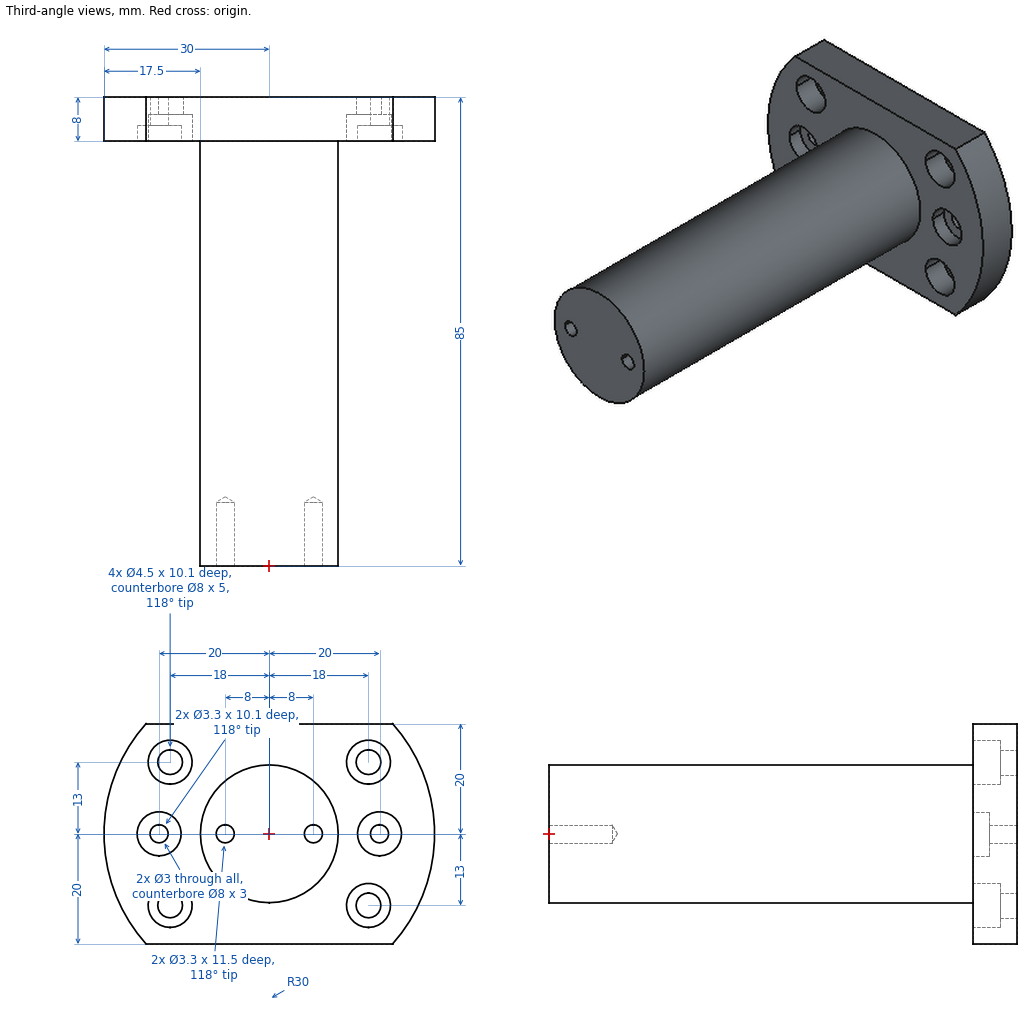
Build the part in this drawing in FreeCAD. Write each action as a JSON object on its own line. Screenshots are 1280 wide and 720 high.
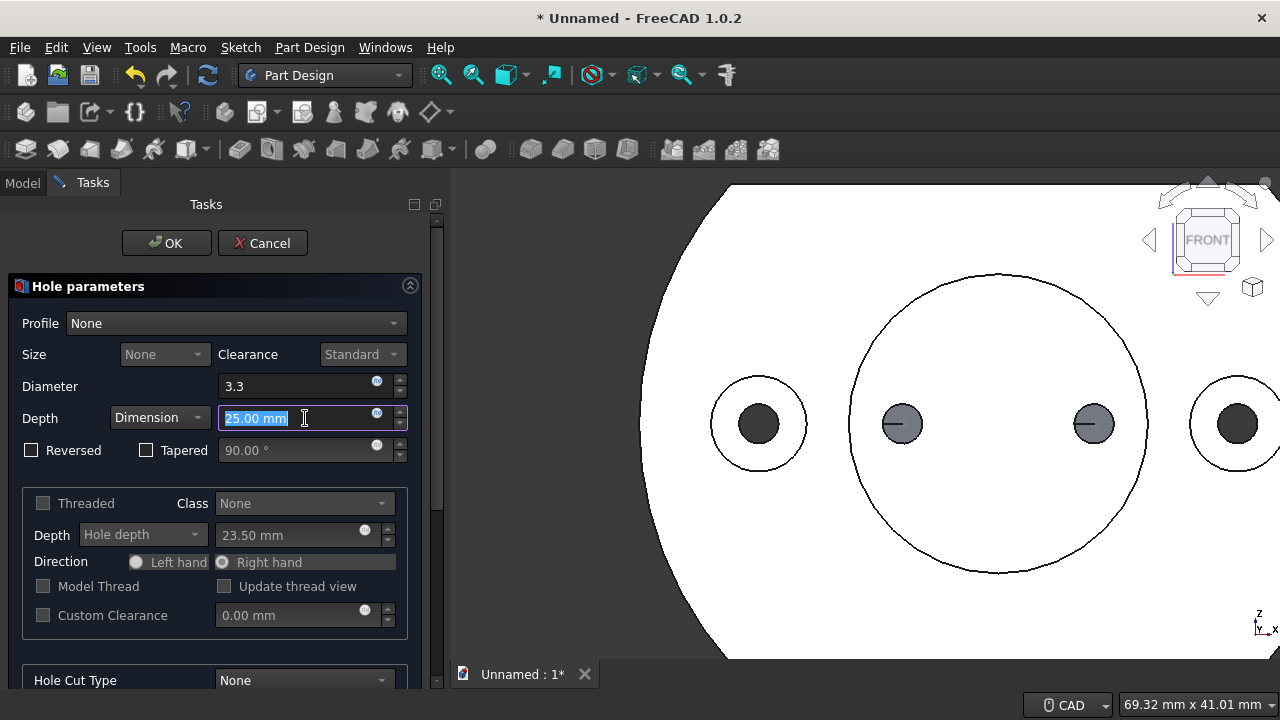
{"action": "type", "text": "10.1"}
{"action": "key", "text": "Tab"}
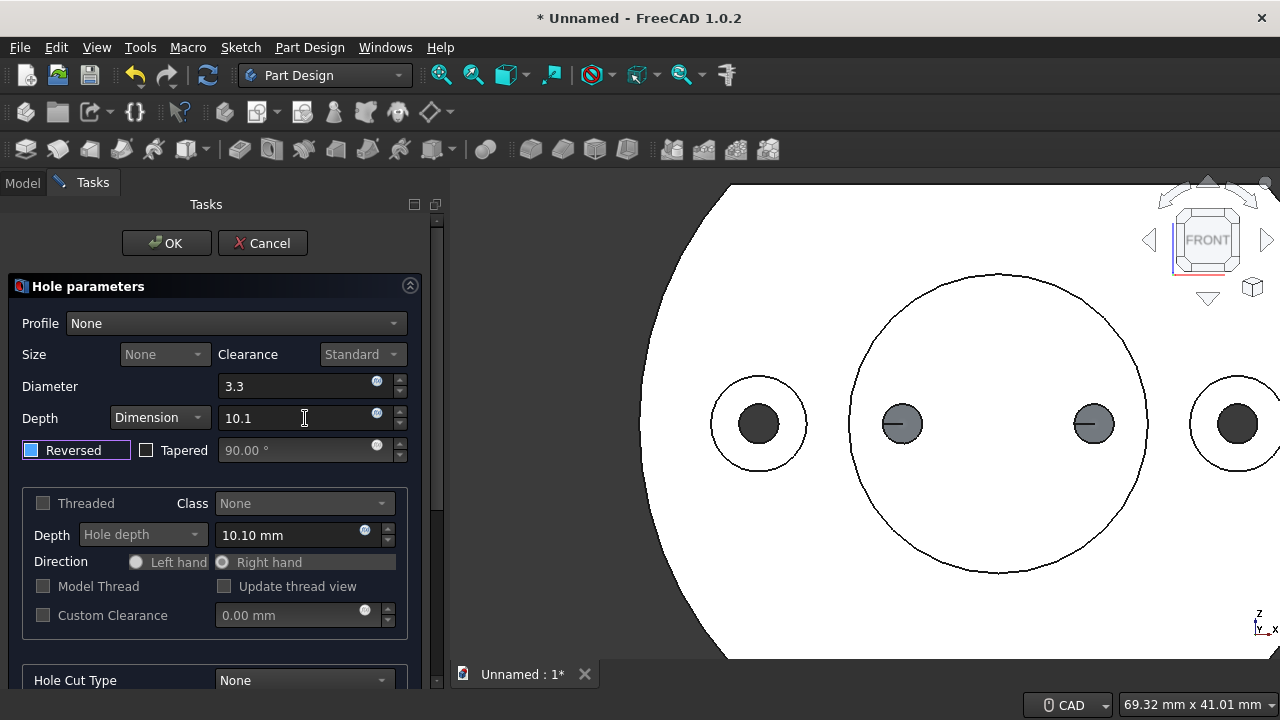
{"action": "left_click", "coordinate": [167, 243]}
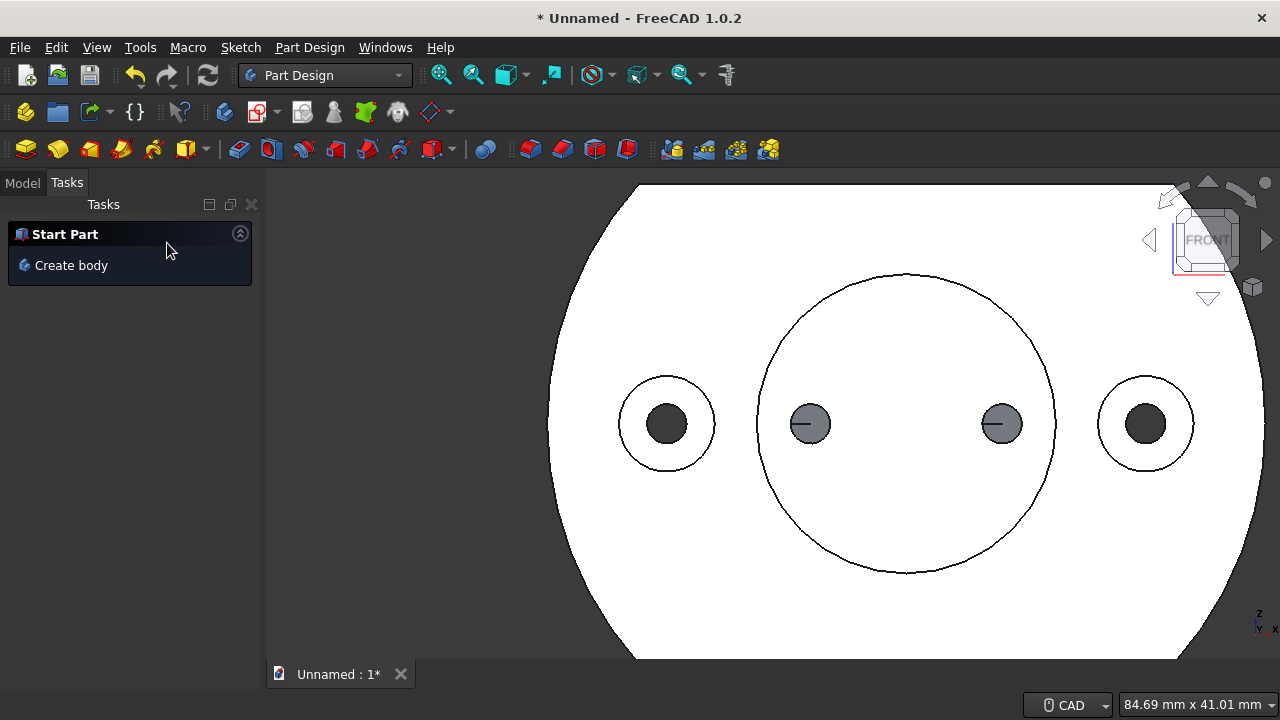
{"action": "left_click", "coordinate": [442, 76]}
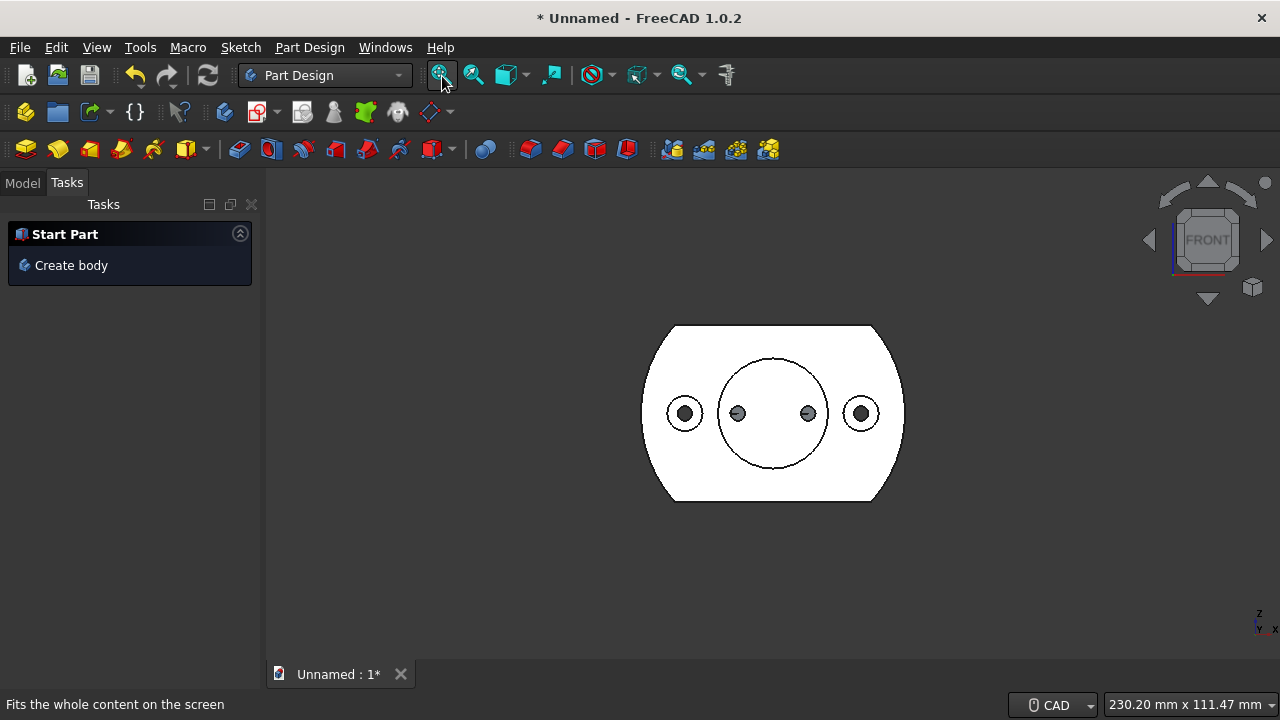
{"action": "left_click", "coordinate": [849, 463]}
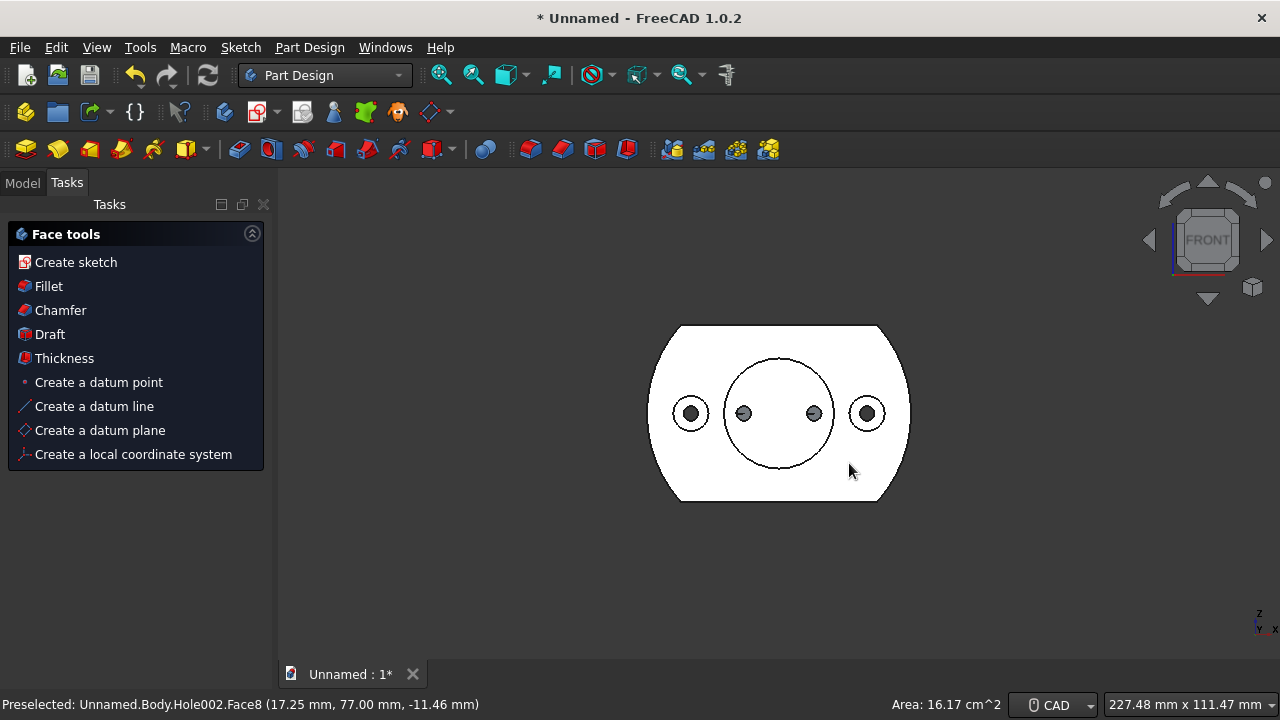
{"action": "left_click", "coordinate": [258, 112]}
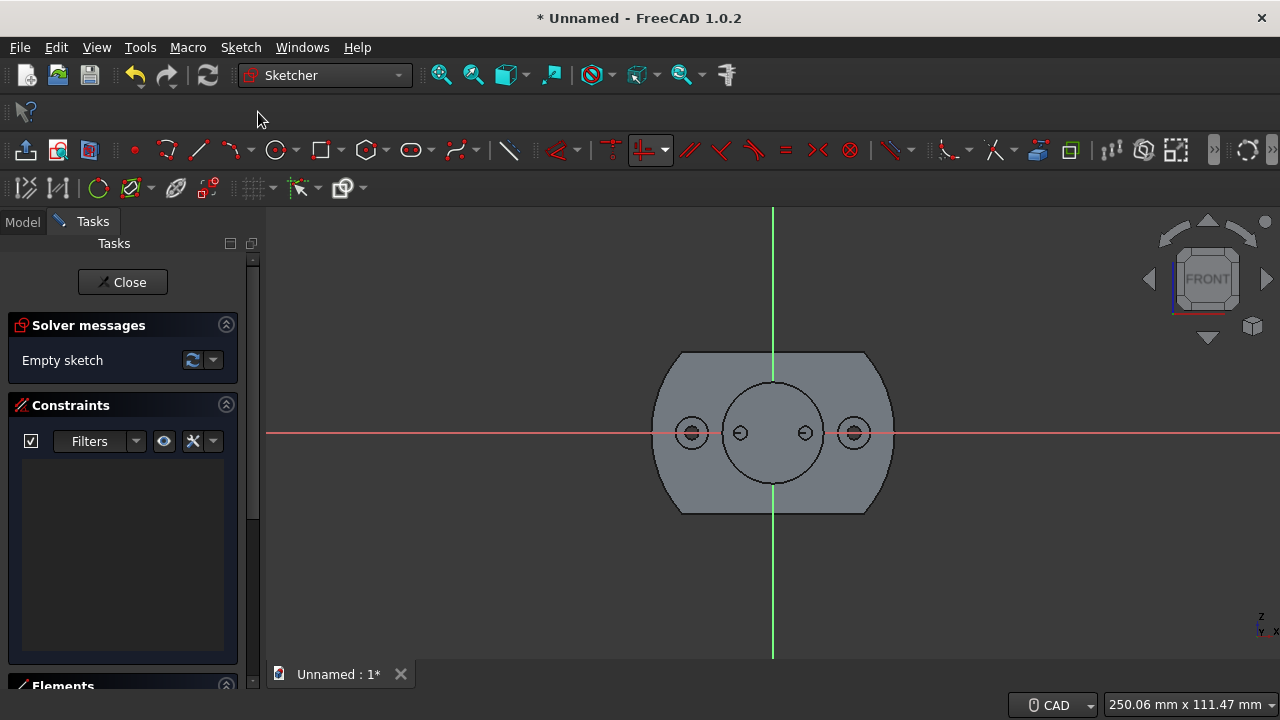
{"action": "scroll", "coordinate": [829, 433], "scroll_direction": "up", "scroll_amount": 4}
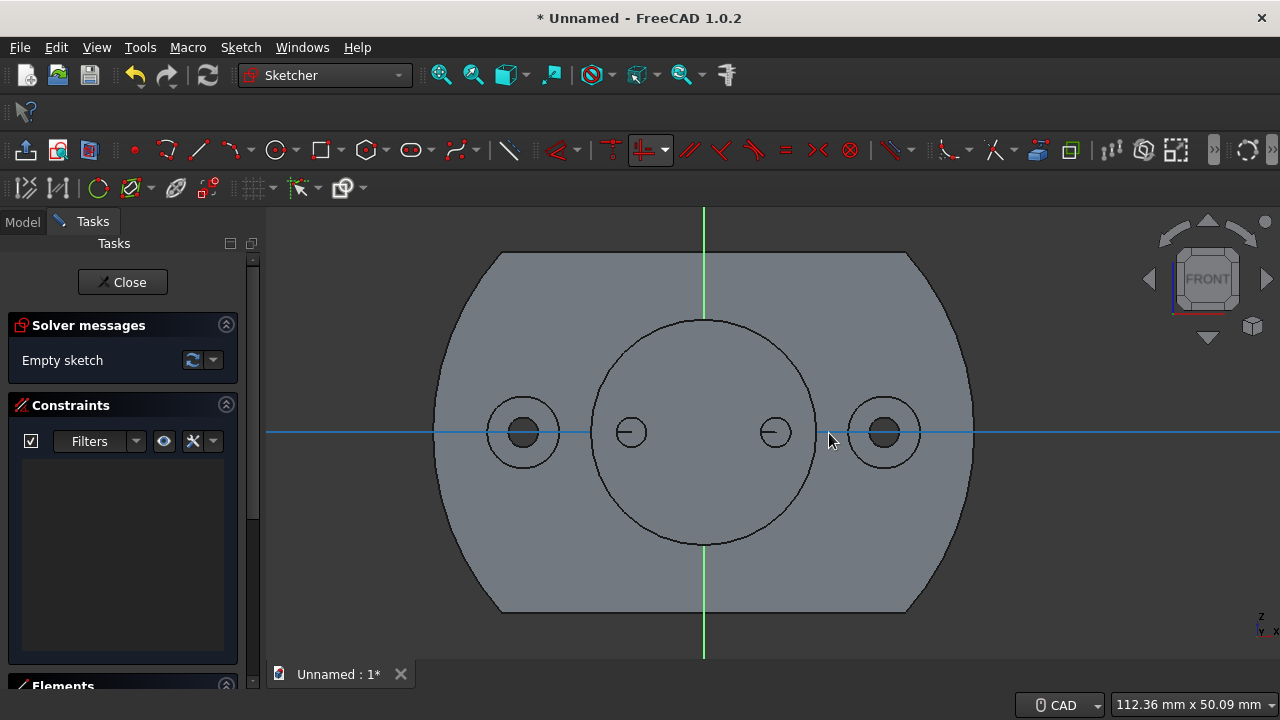
{"action": "left_click", "coordinate": [276, 150]}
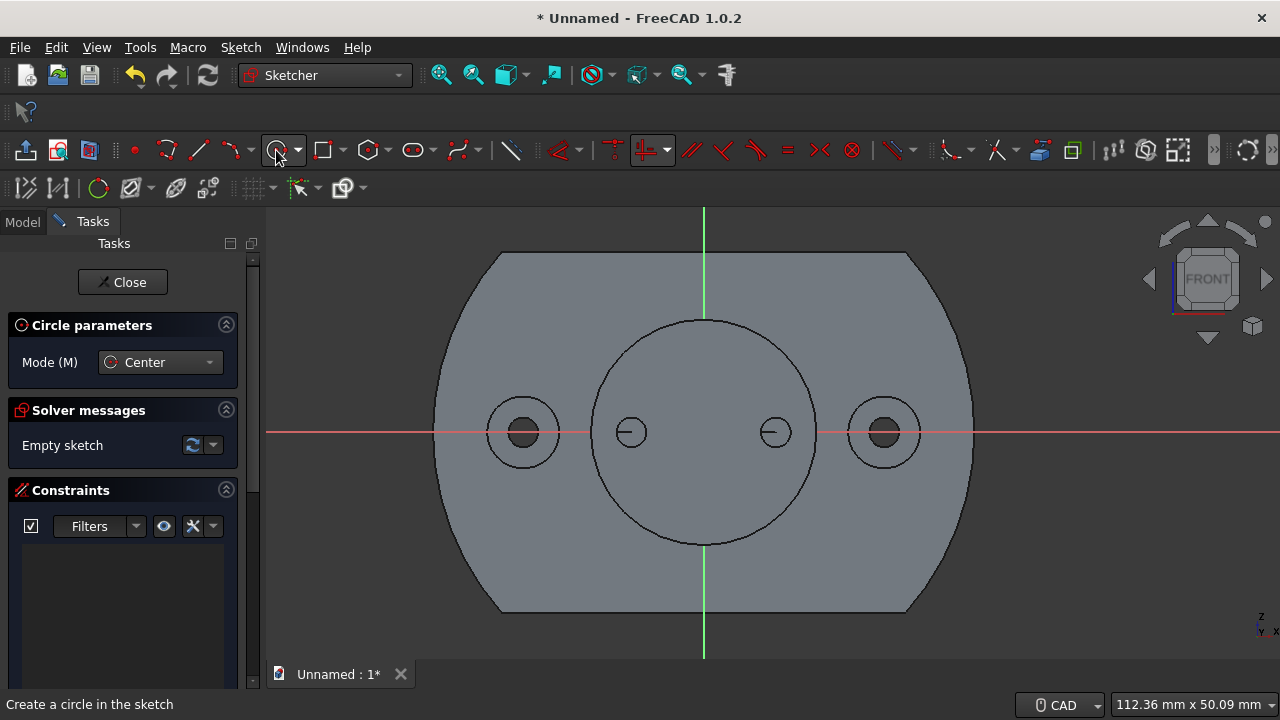
{"action": "left_click", "coordinate": [541, 315]}
{"action": "mouse_move", "coordinate": [556, 301]}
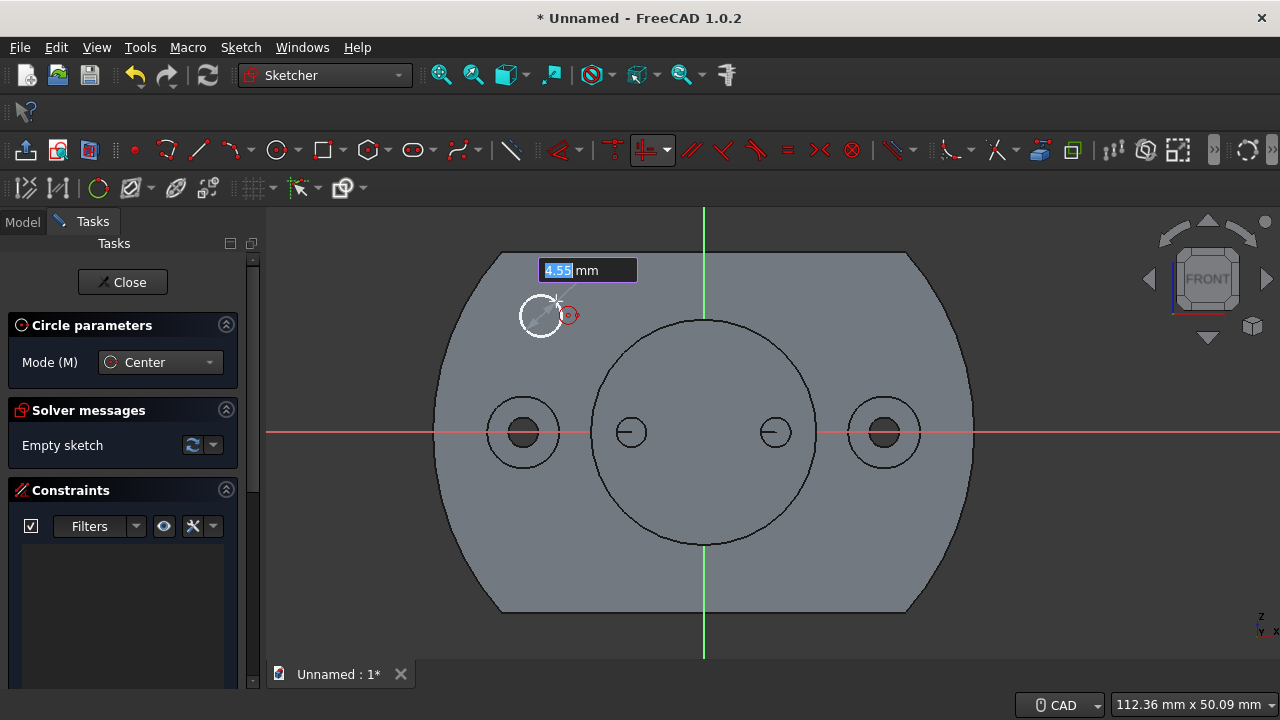
{"action": "type", "text": "4.5"}
{"action": "key", "text": "Return"}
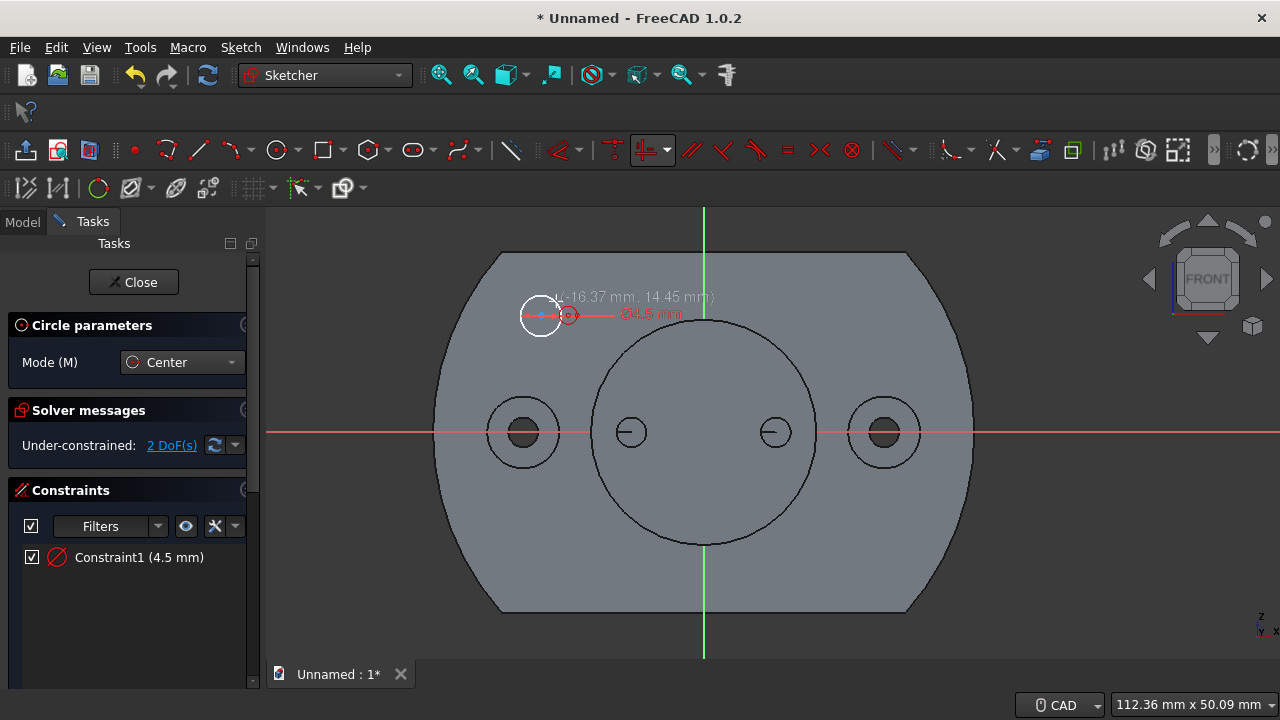
{"action": "left_click", "coordinate": [866, 315]}
{"action": "mouse_move", "coordinate": [880, 301]}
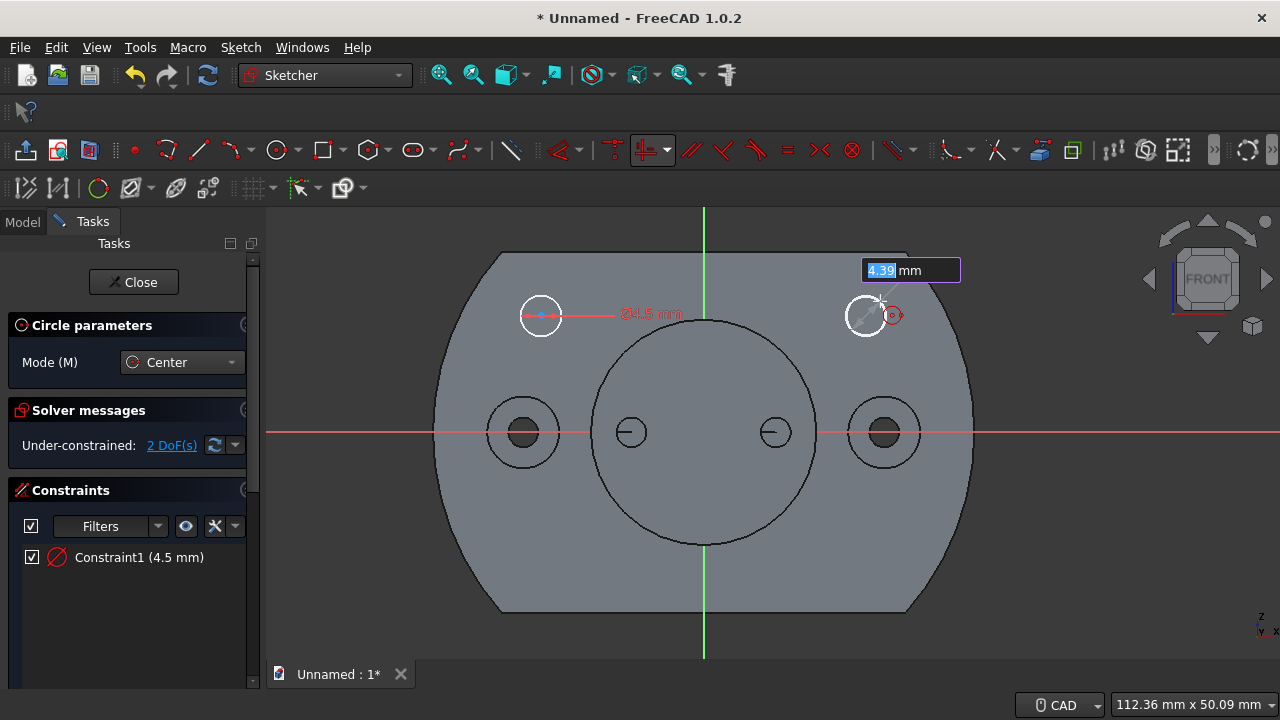
{"action": "type", "text": "4.5"}
{"action": "key", "text": "Return"}